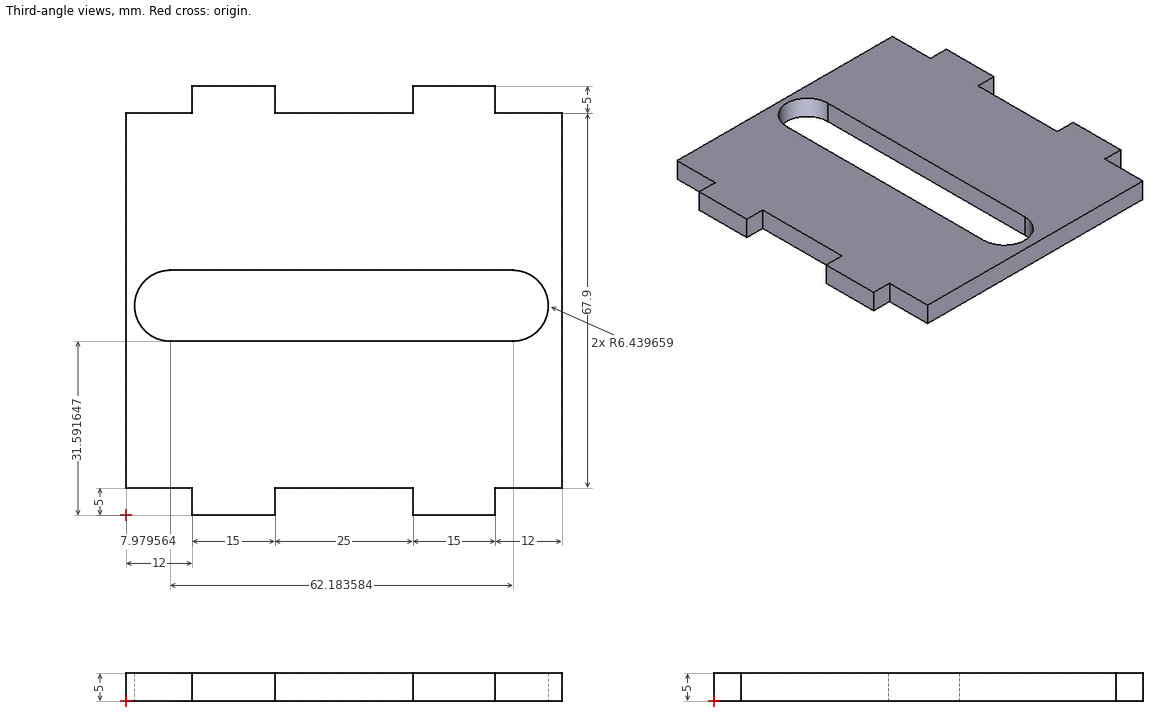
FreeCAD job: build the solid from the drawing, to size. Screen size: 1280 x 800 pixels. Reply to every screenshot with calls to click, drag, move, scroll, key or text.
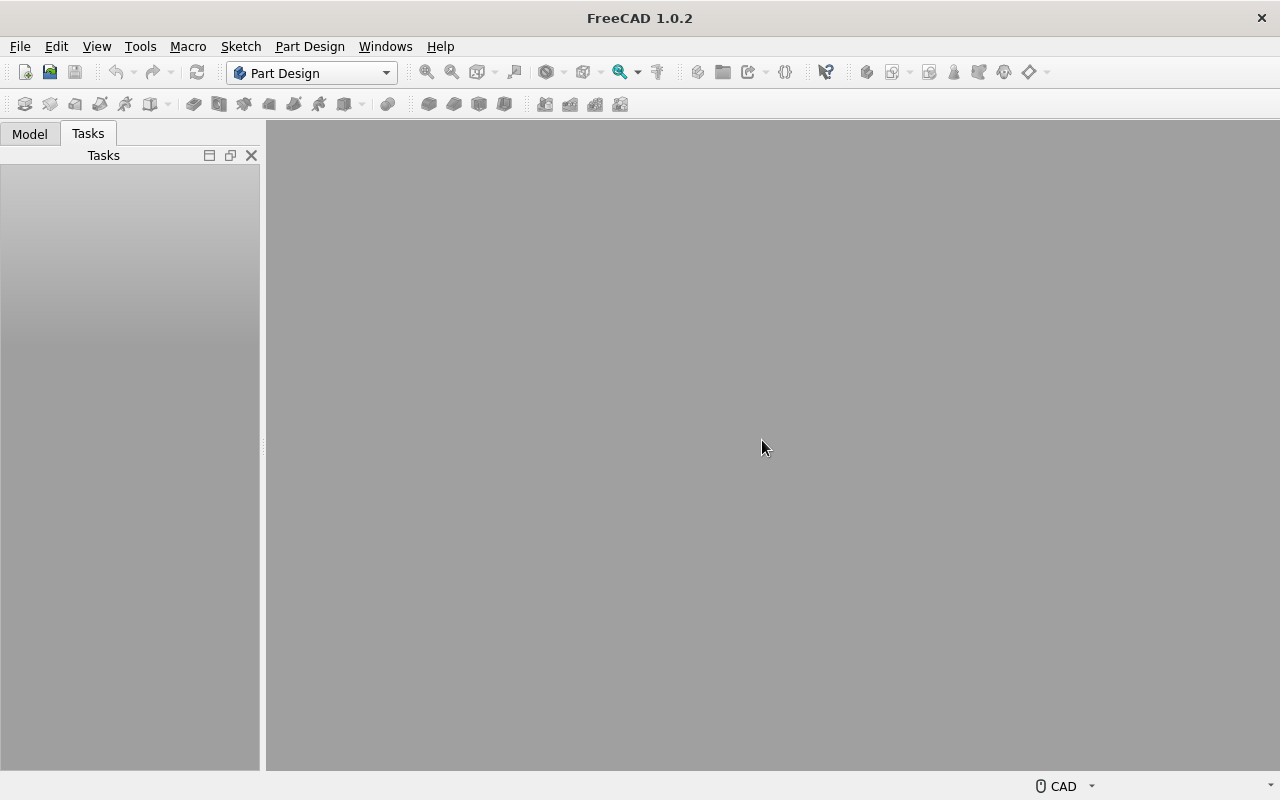
click(25, 72)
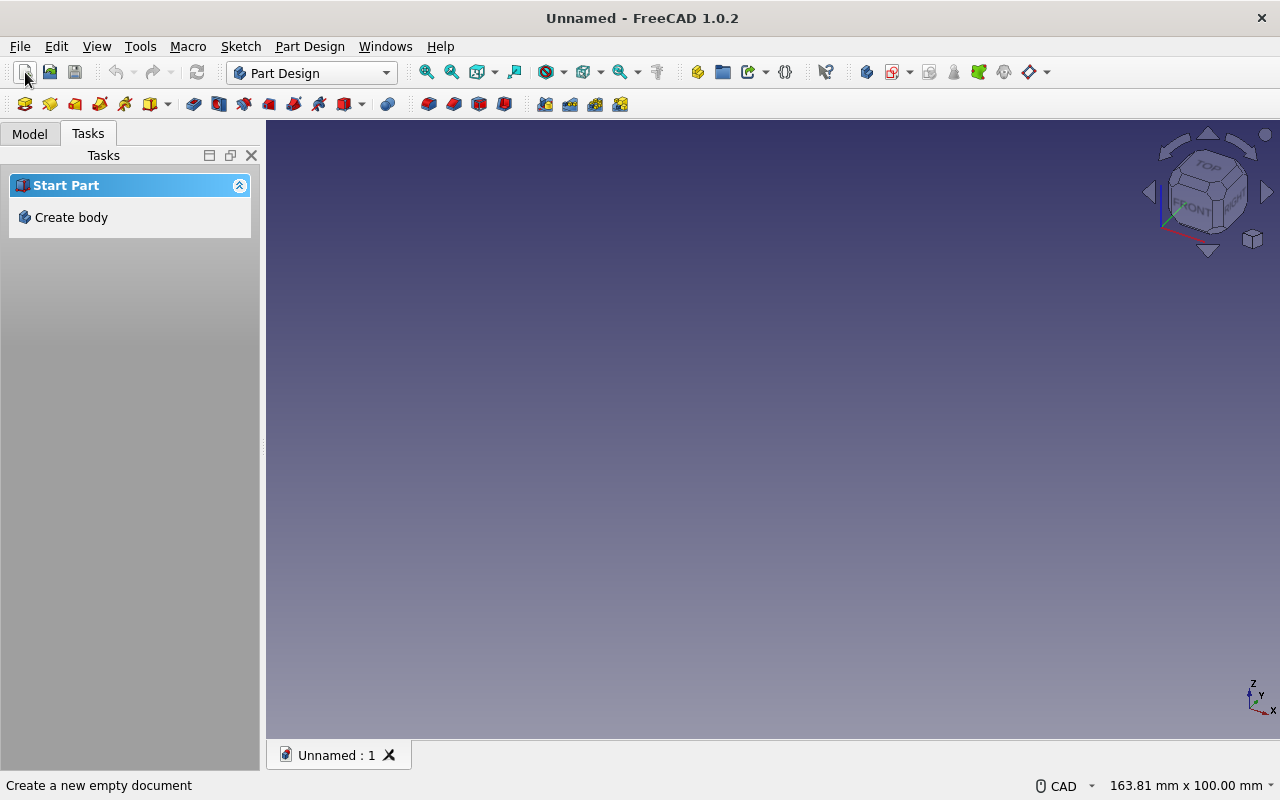
click(892, 72)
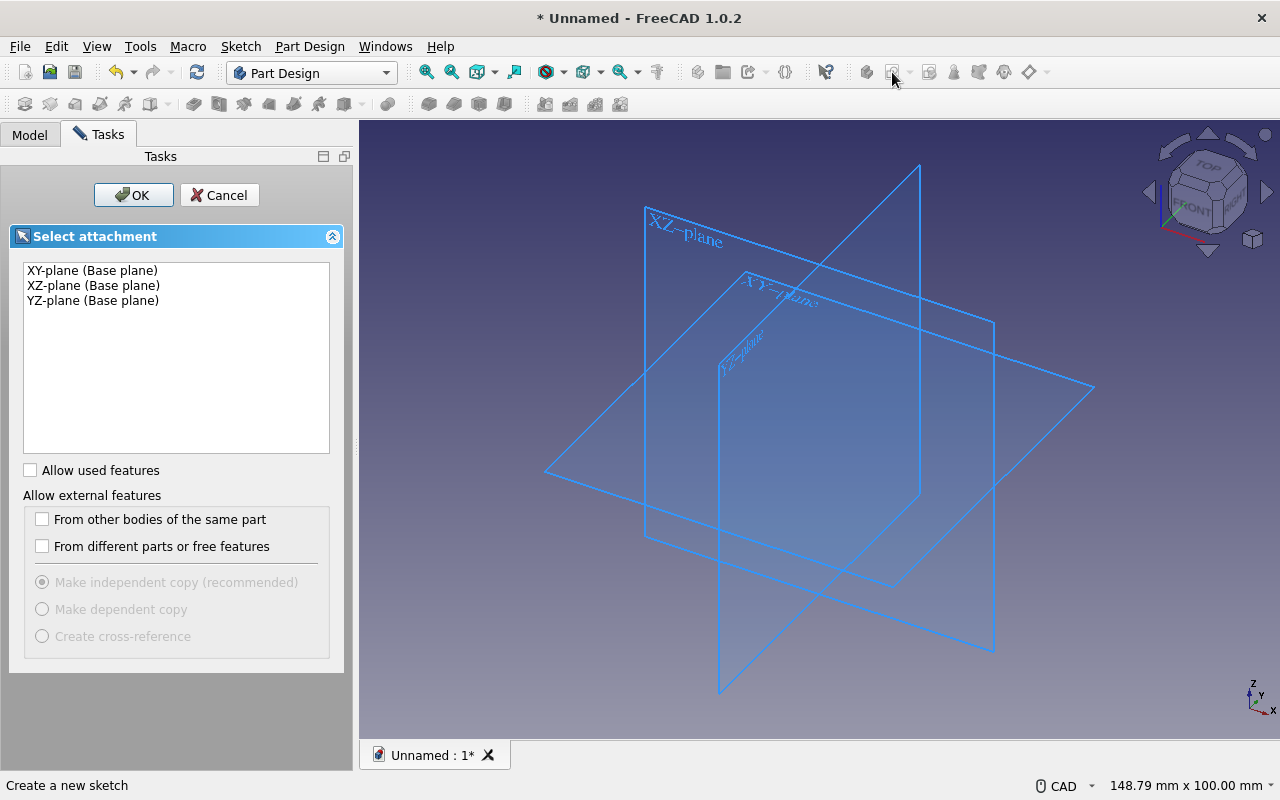
click(84, 270)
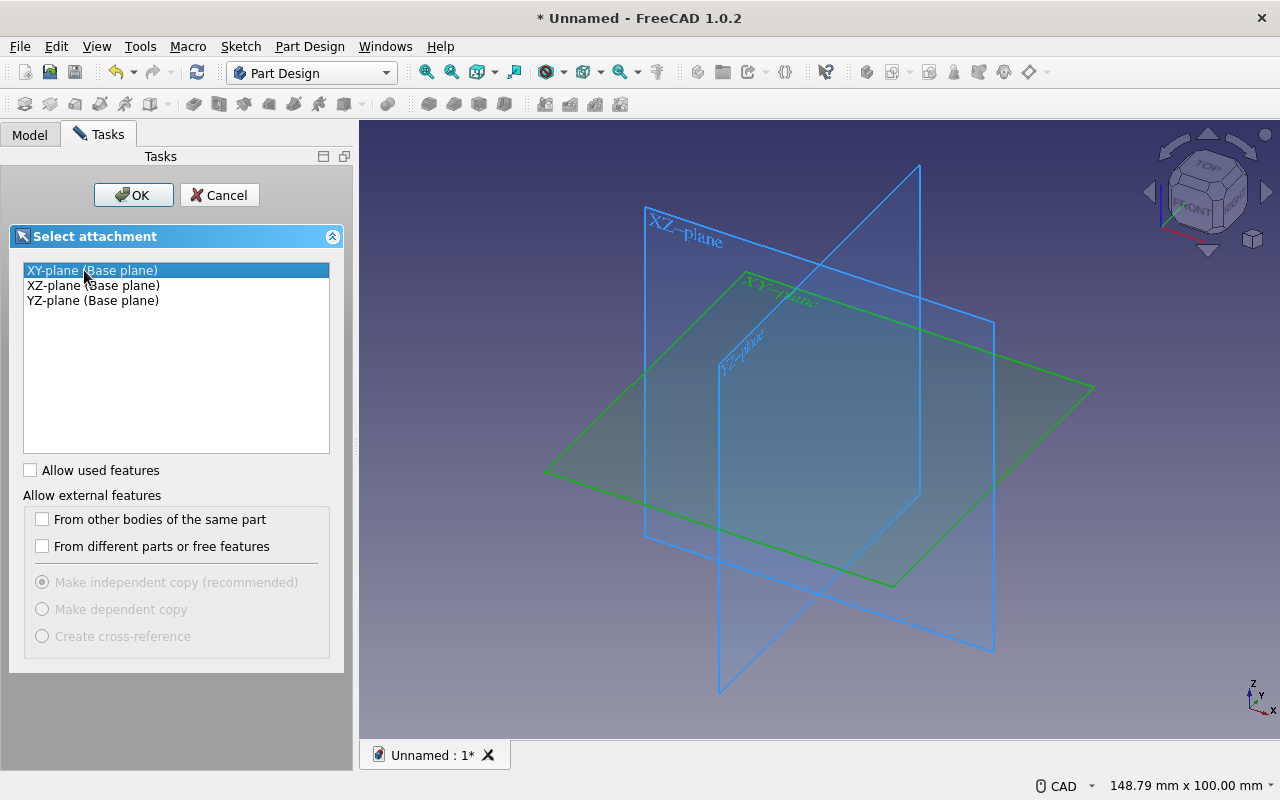
click(134, 195)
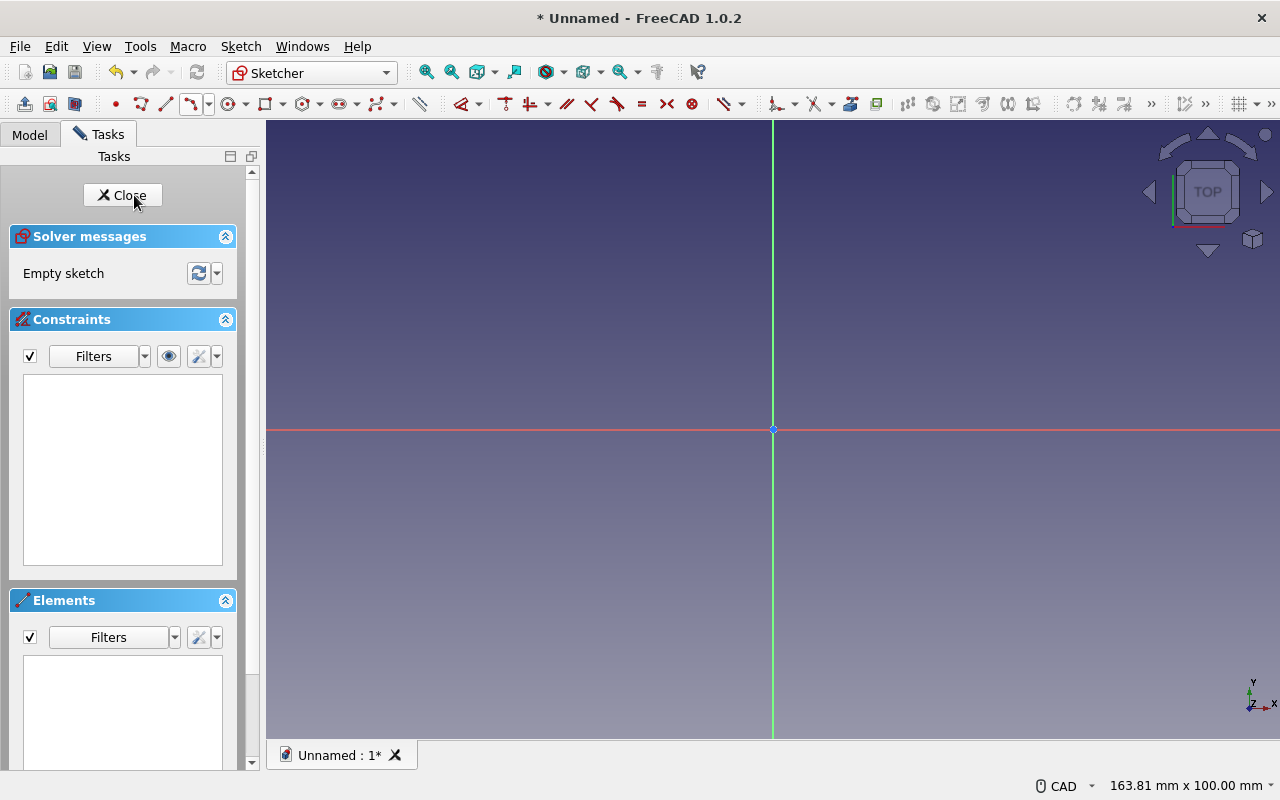
scroll(294, 711, down, 2)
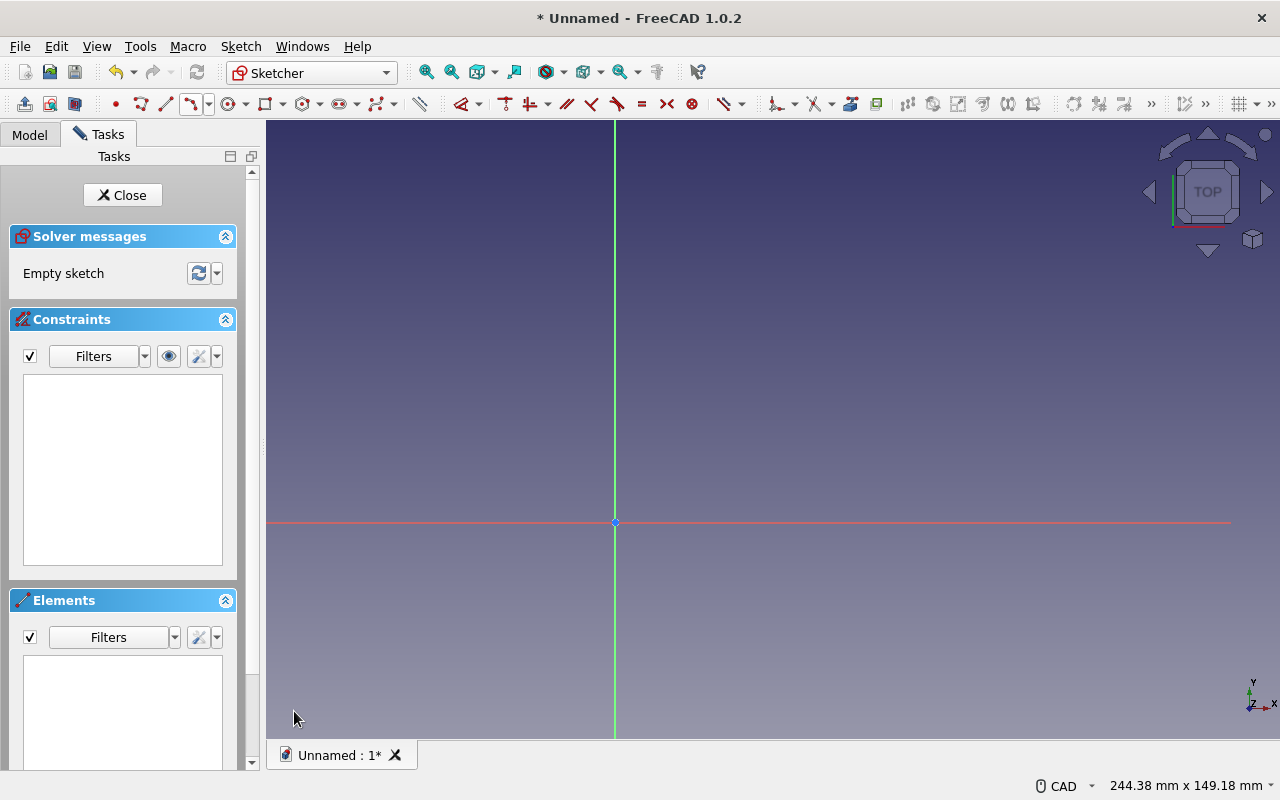
click(141, 104)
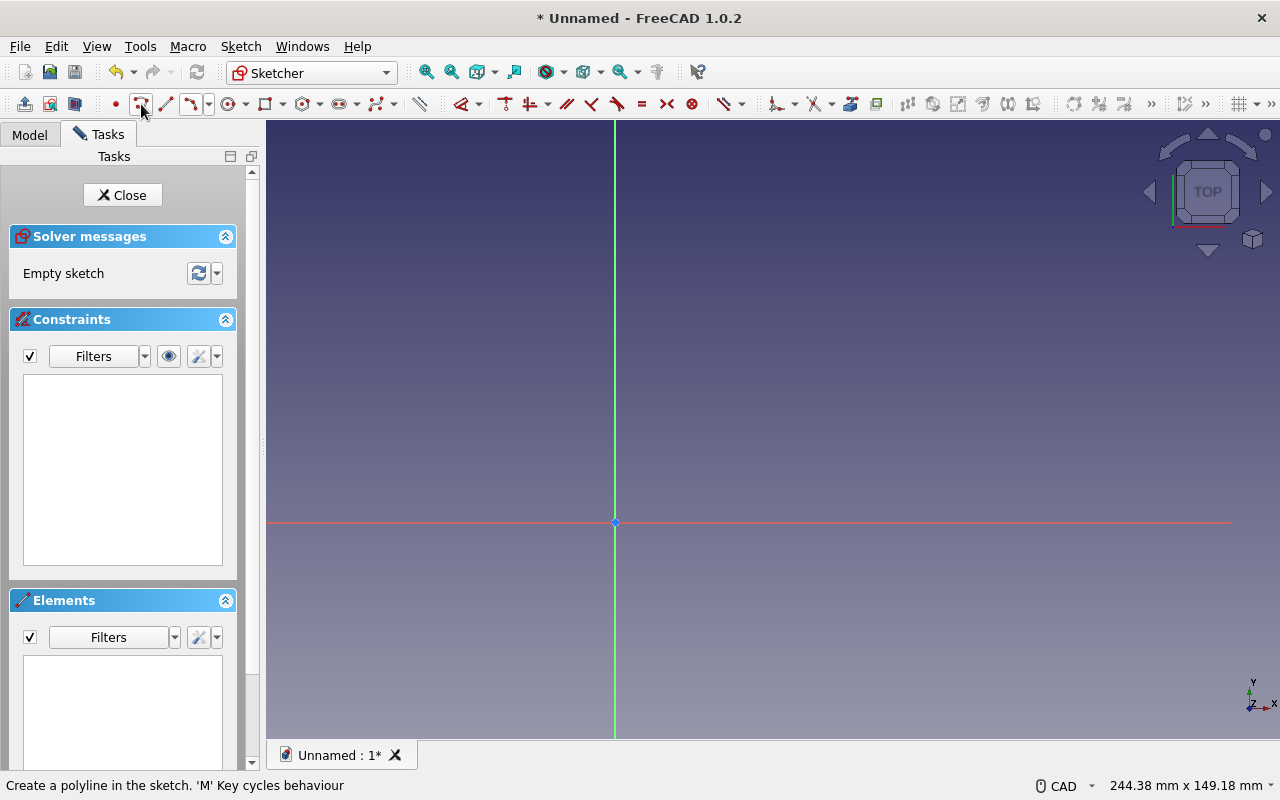
click(615, 502)
click(665, 502)
click(665, 523)
click(727, 514)
click(727, 502)
click(831, 502)
click(831, 523)
click(893, 514)
click(893, 502)
click(943, 502)
click(943, 220)
click(893, 220)
click(893, 199)
click(831, 199)
click(831, 220)
click(727, 220)
click(727, 199)
click(665, 199)
click(665, 220)
click(624, 220)
click(615, 503)
key(Escape)
key(Escape)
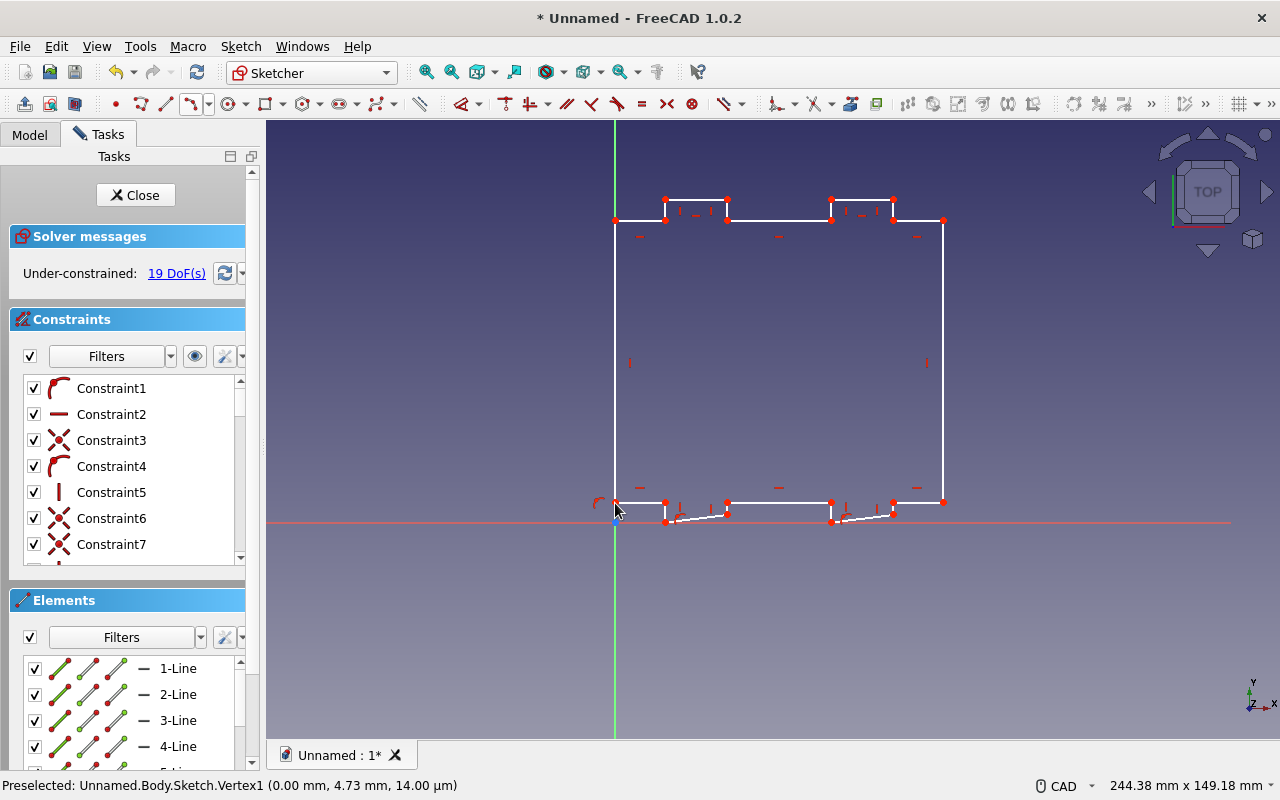
click(690, 520)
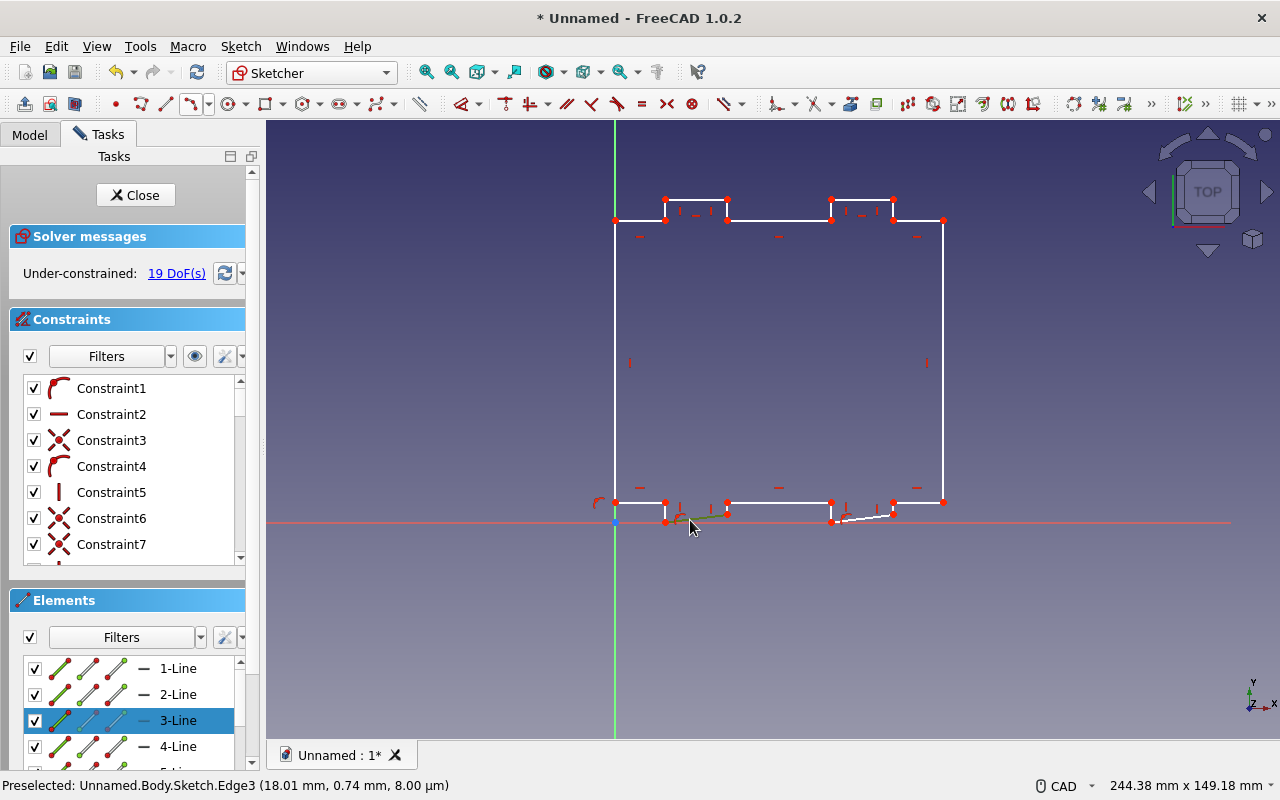
key(h)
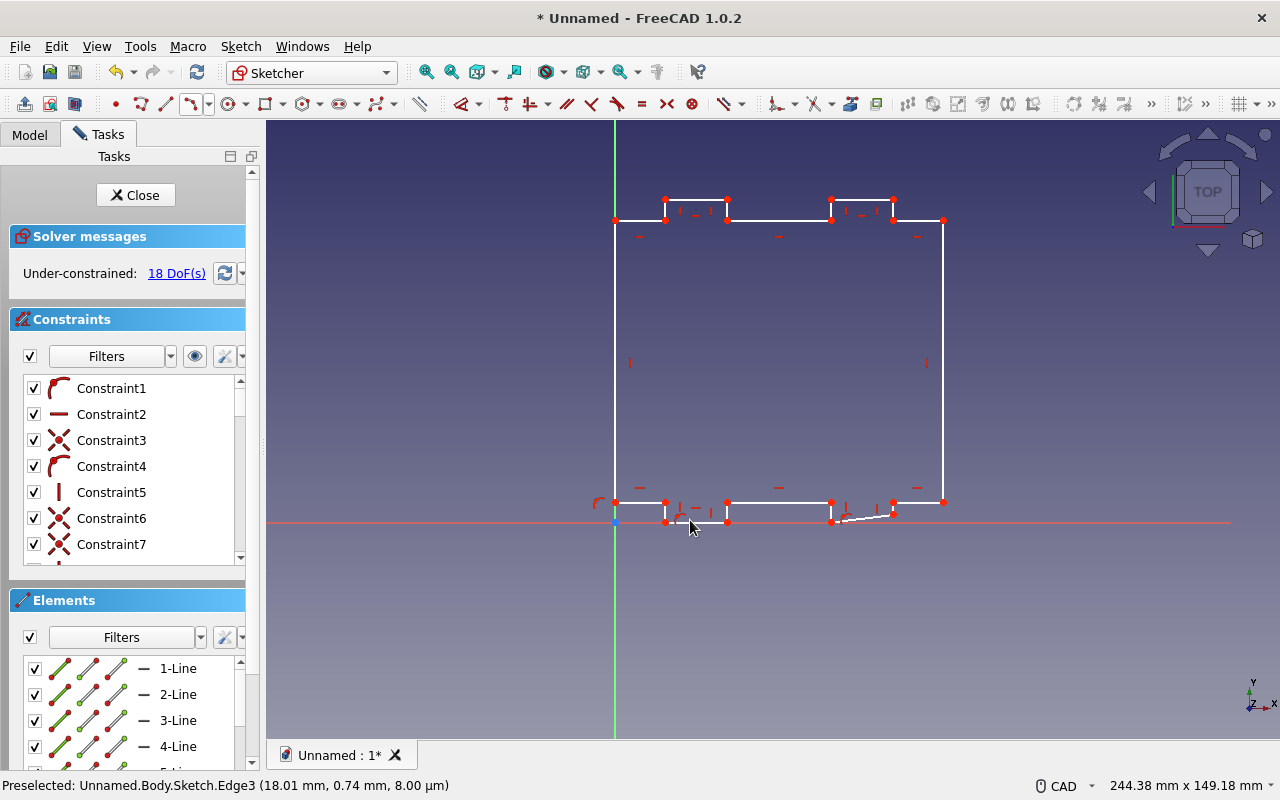
click(856, 520)